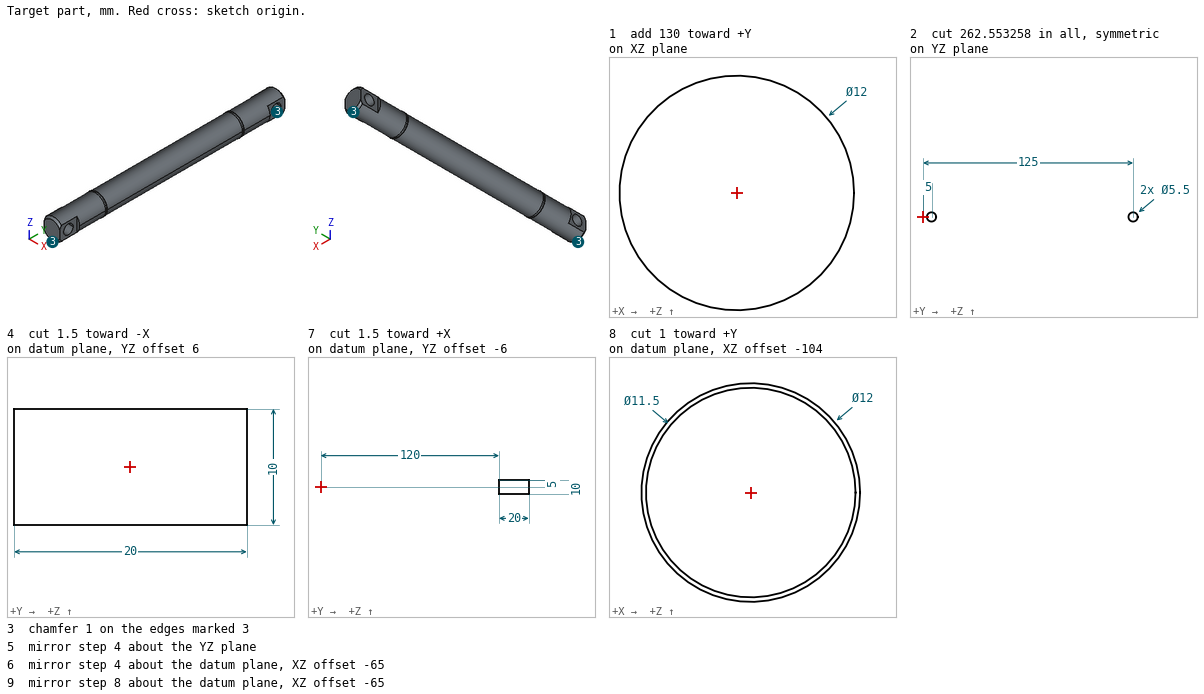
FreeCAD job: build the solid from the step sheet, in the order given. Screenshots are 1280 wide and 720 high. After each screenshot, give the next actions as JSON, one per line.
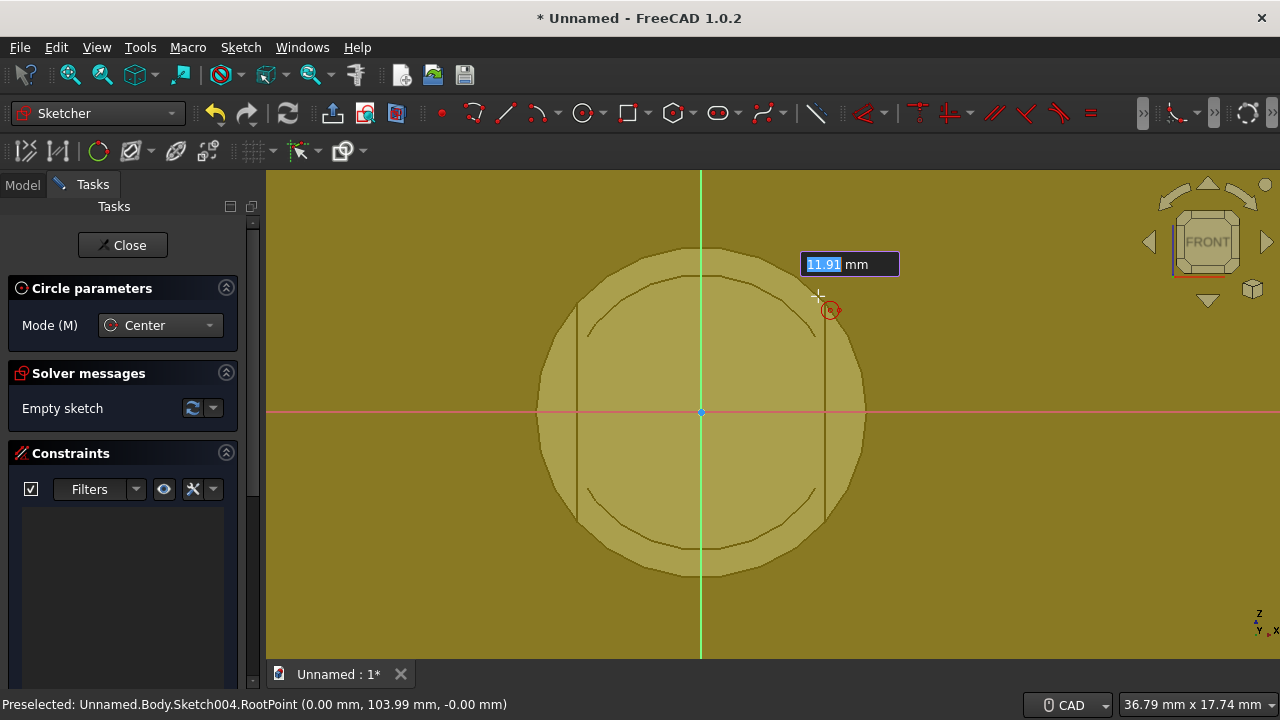
{"action": "type", "text": "12"}
{"action": "key", "text": "Return"}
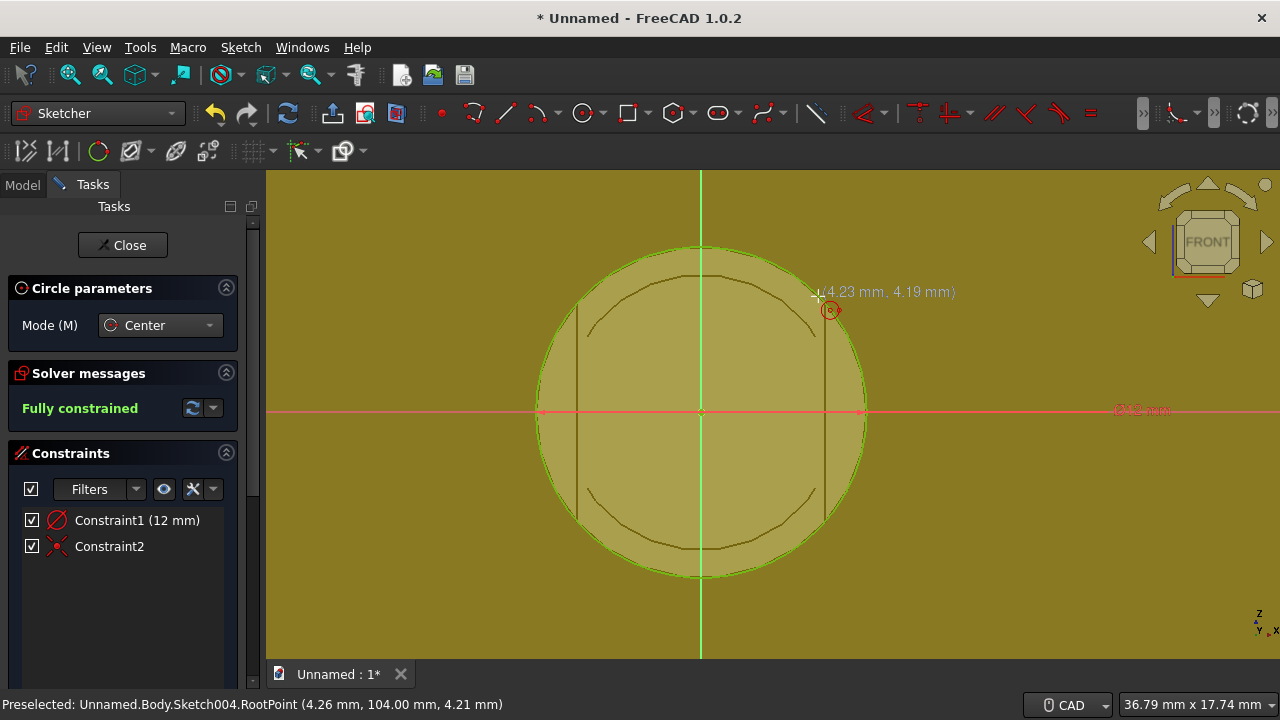
{"action": "left_click", "coordinate": [701, 412]}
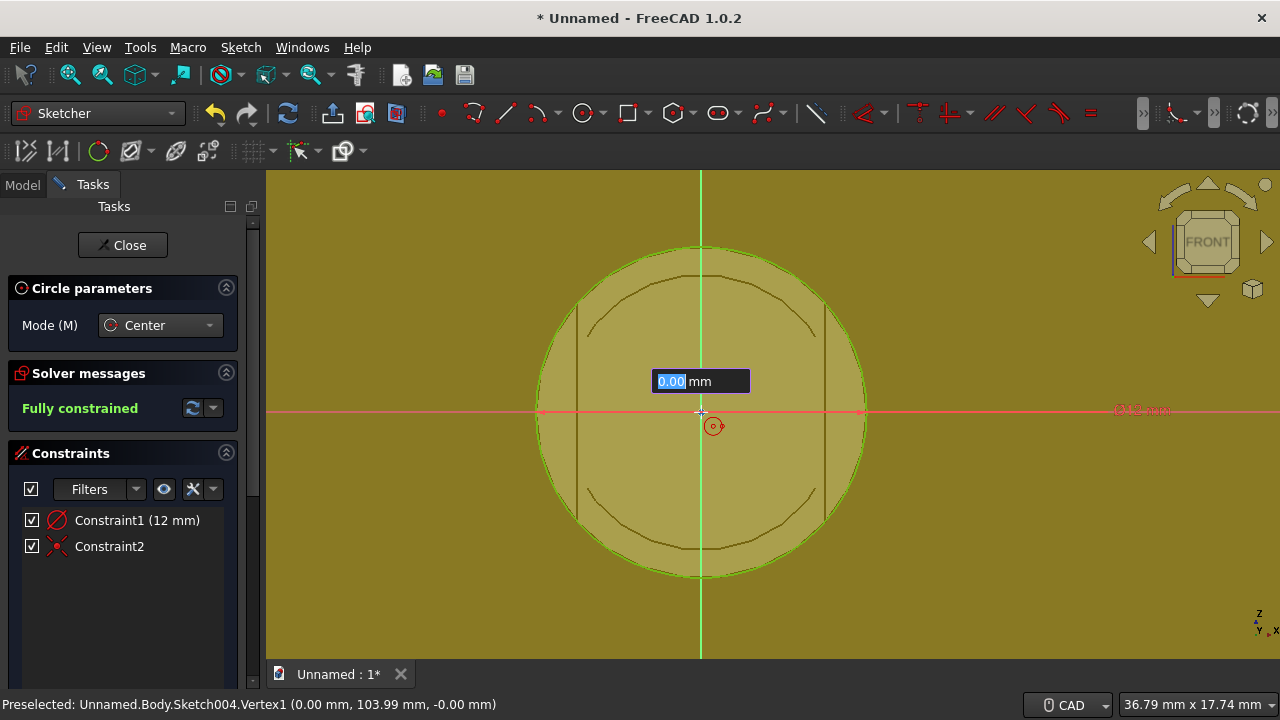
{"action": "scroll", "coordinate": [756, 264], "scroll_direction": "up", "scroll_amount": 5}
{"action": "mouse_move", "coordinate": [754, 262]}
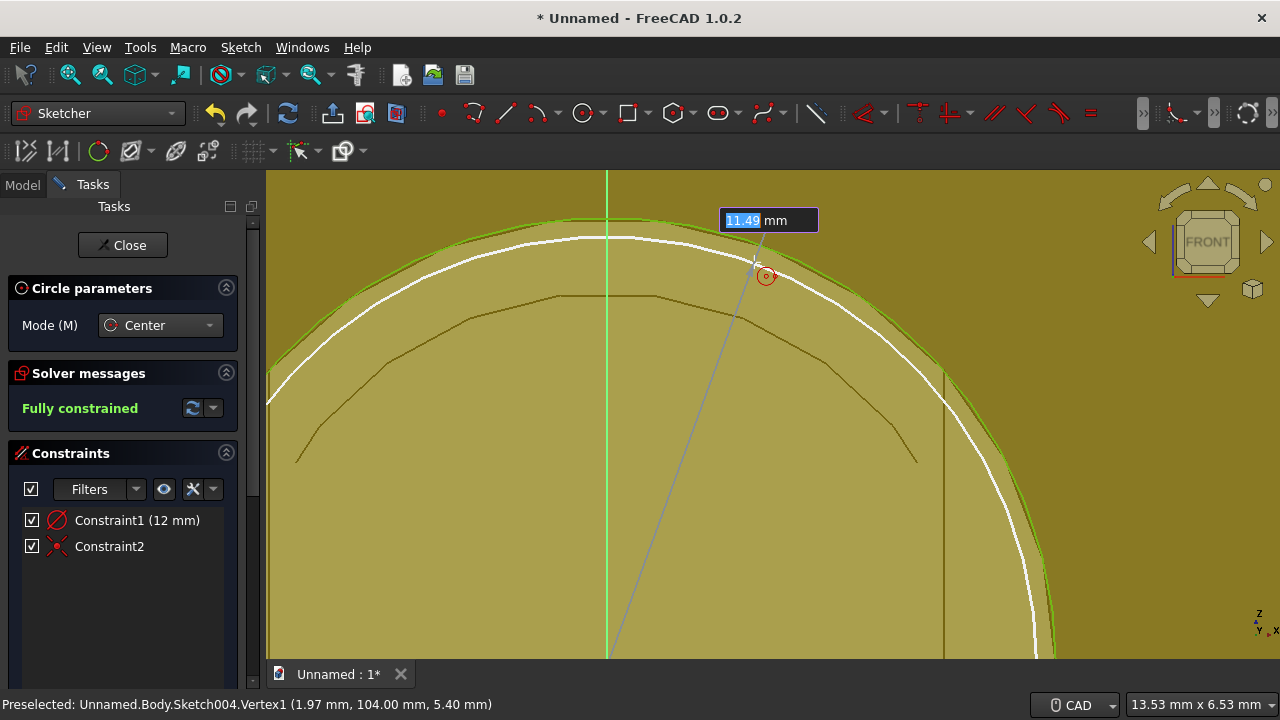
{"action": "type", "text": "11.5"}
{"action": "key", "text": "Return"}
{"action": "key", "text": "Escape"}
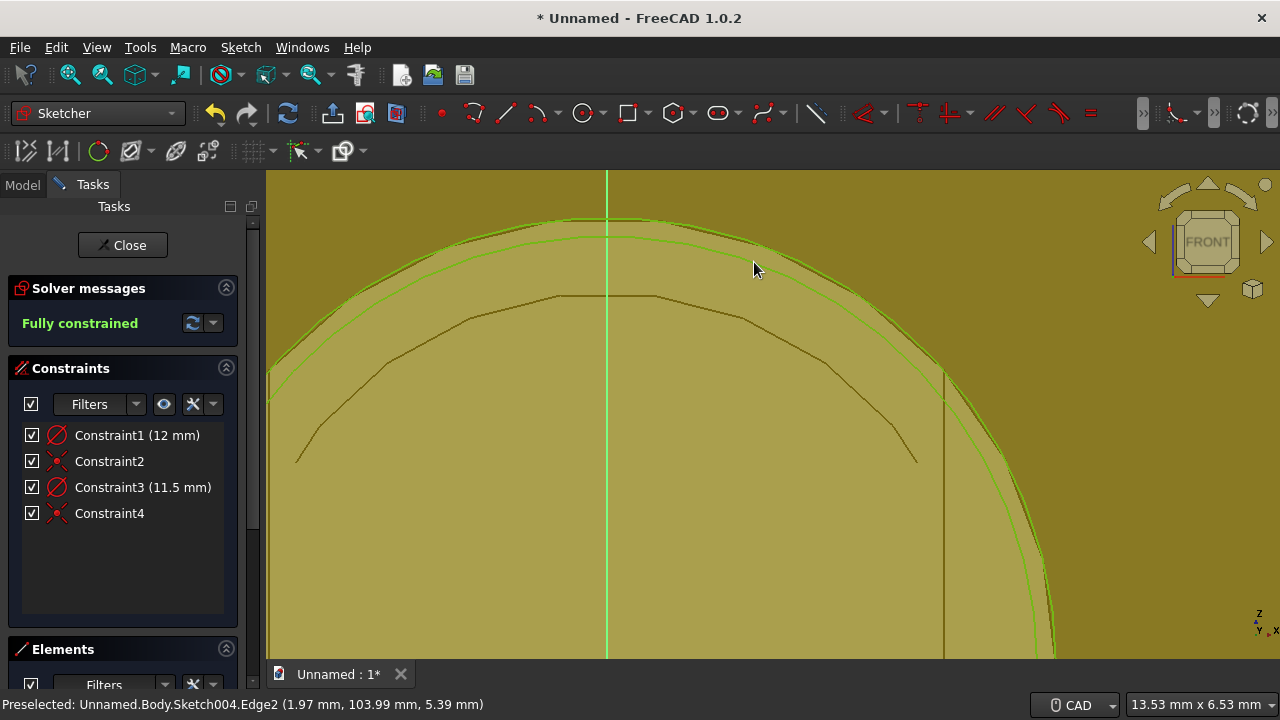
{"action": "left_click", "coordinate": [123, 245]}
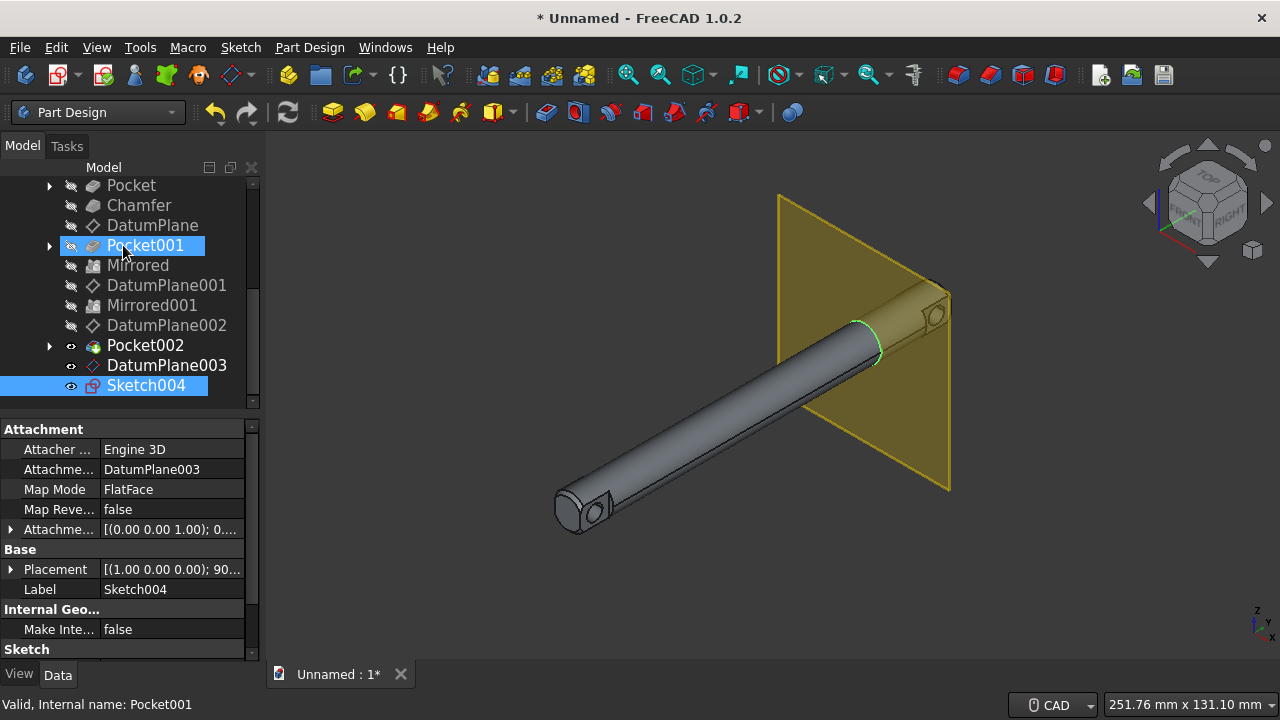
{"action": "left_click", "coordinate": [548, 112]}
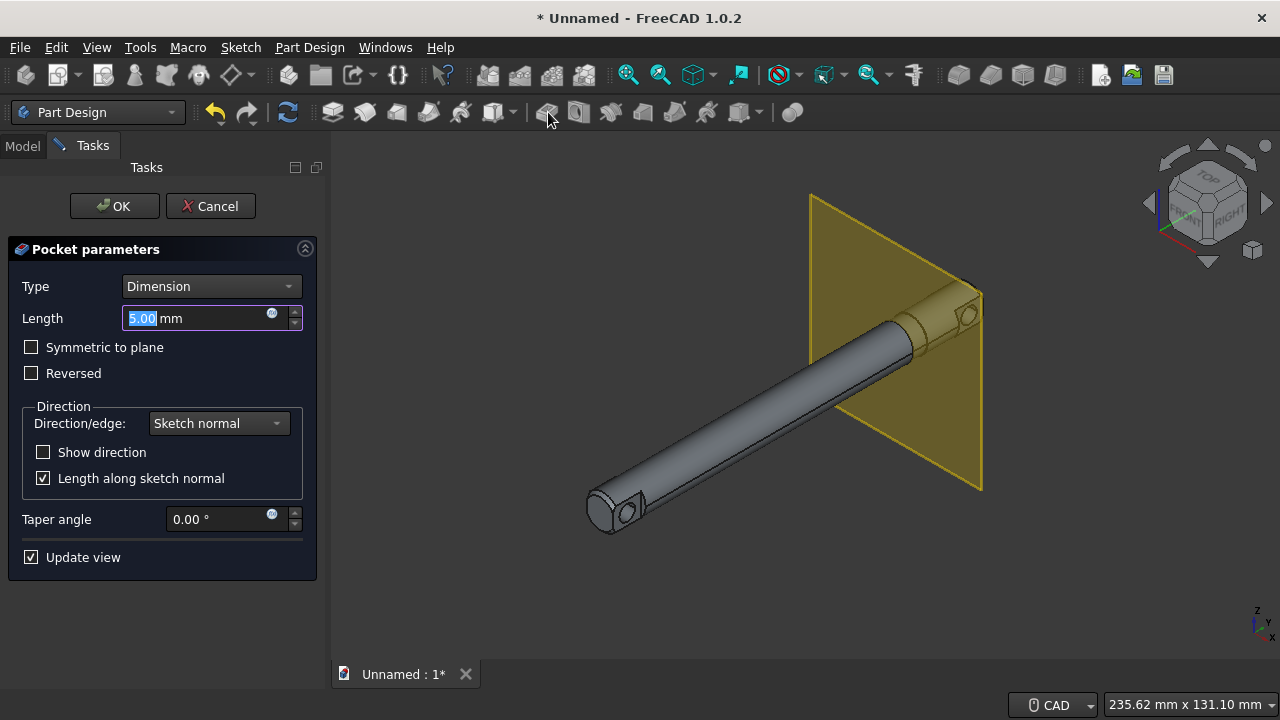
{"action": "type", "text": "1"}
{"action": "key", "text": "Tab"}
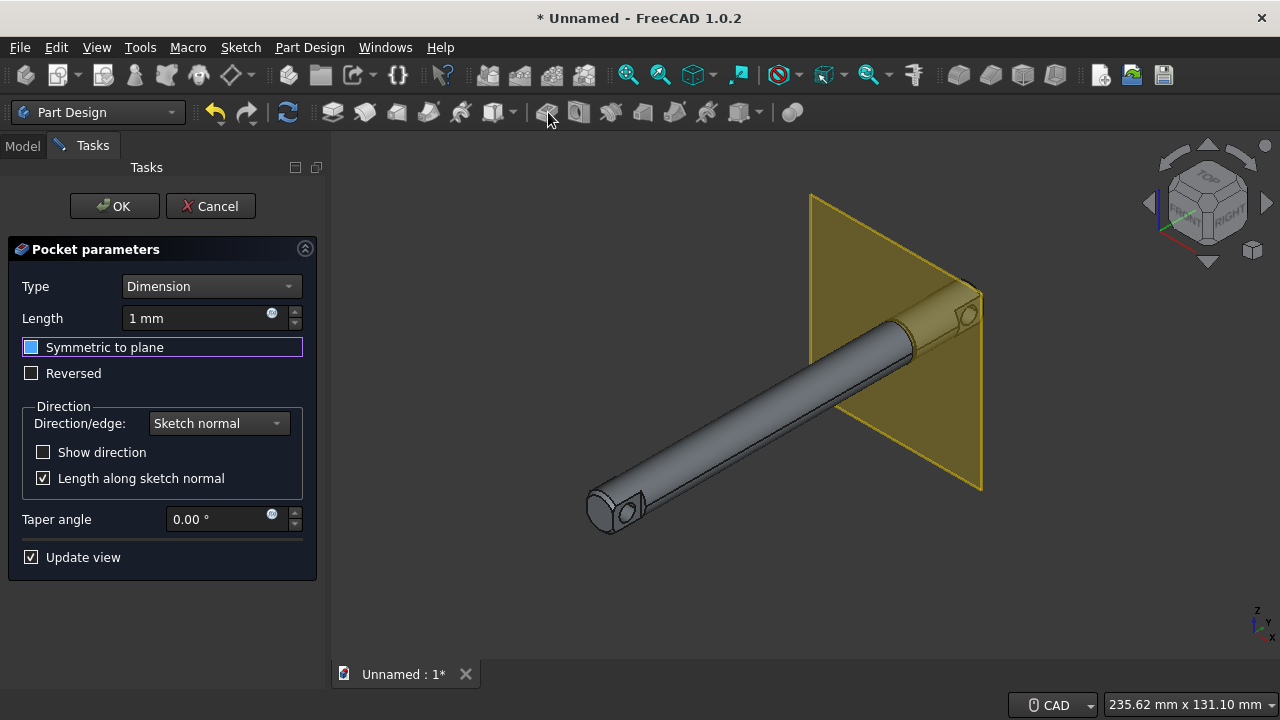
{"action": "left_click", "coordinate": [115, 206]}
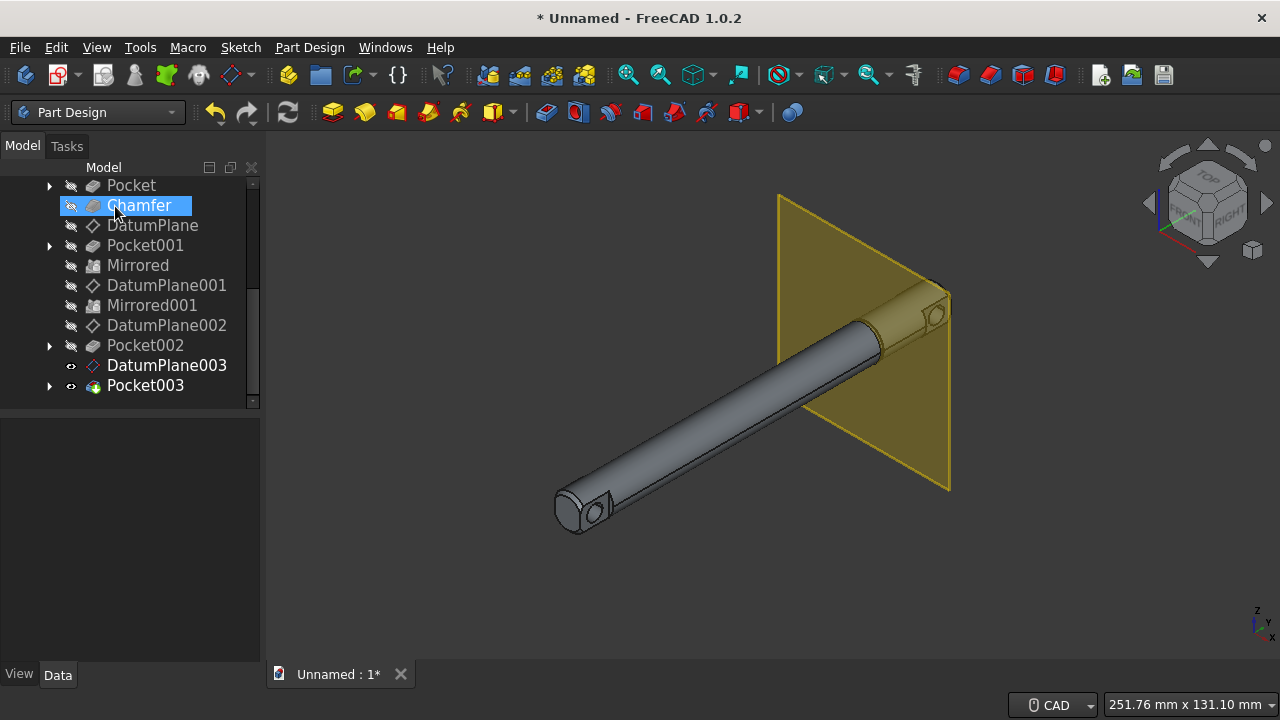
{"action": "left_click", "coordinate": [116, 366]}
{"action": "key", "text": "space"}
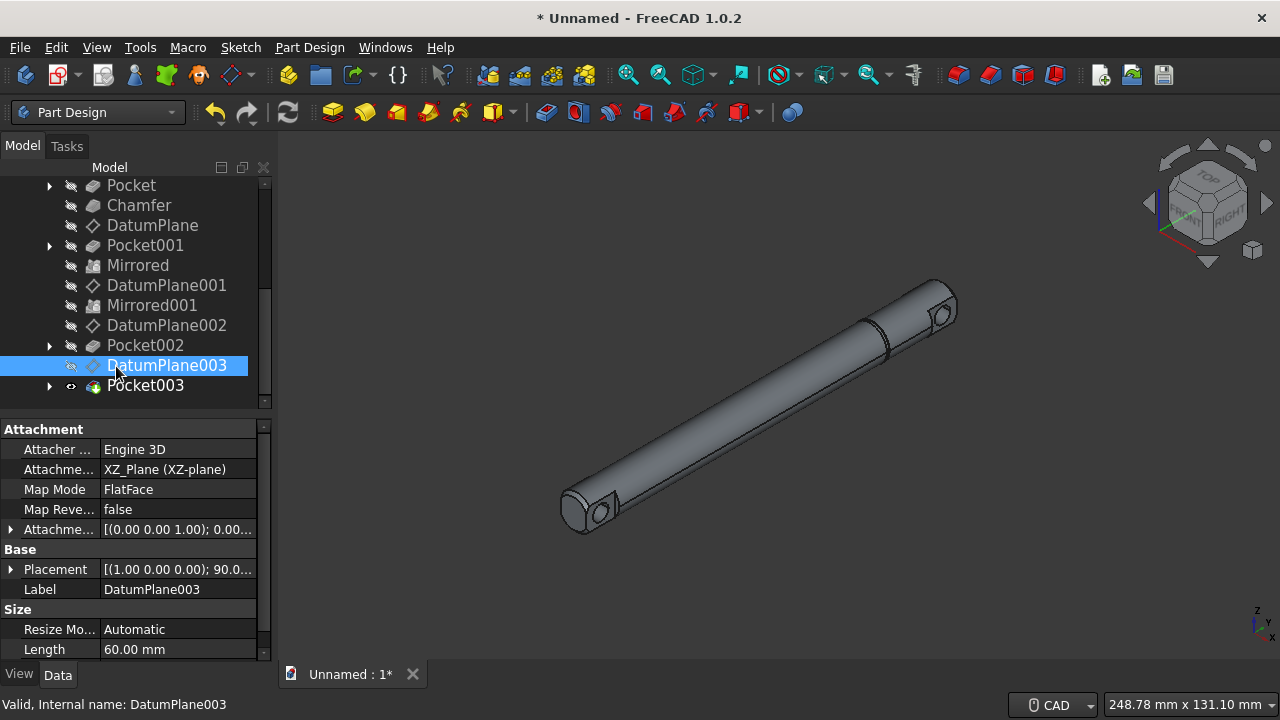
{"action": "scroll", "coordinate": [140, 281], "scroll_direction": "down", "scroll_amount": 3}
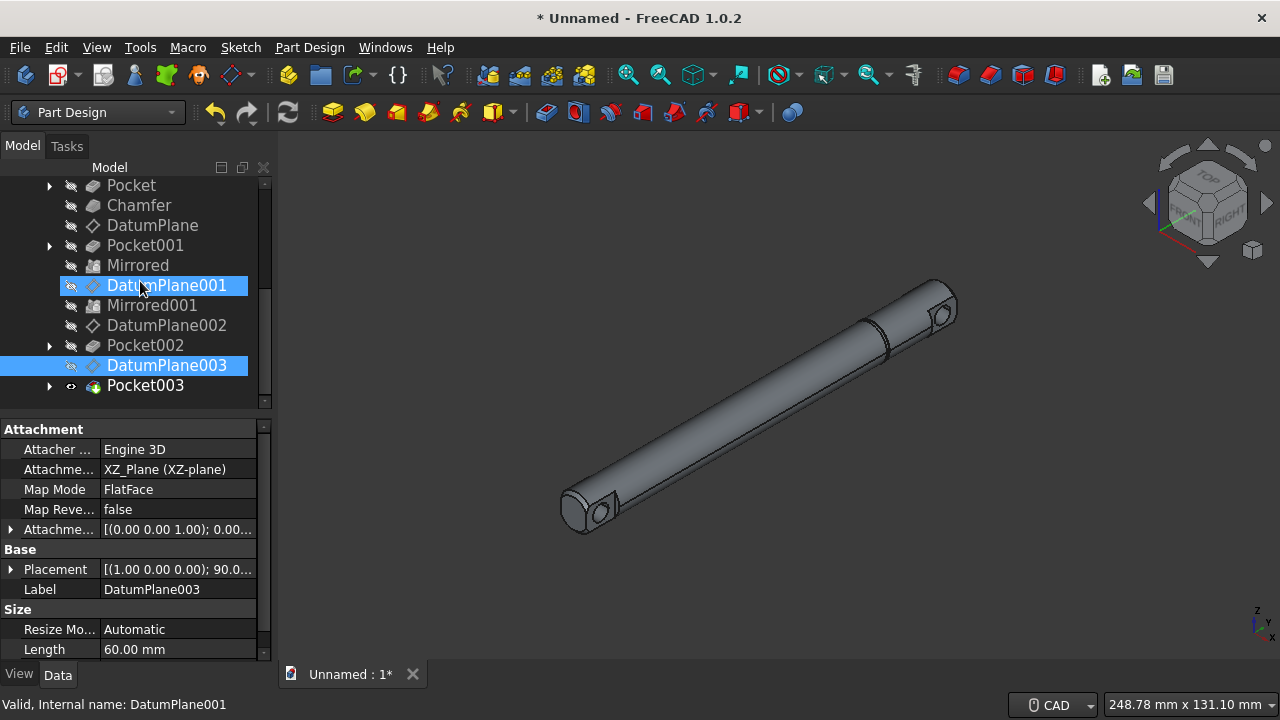
{"action": "scroll", "coordinate": [140, 281], "scroll_direction": "up", "scroll_amount": 15}